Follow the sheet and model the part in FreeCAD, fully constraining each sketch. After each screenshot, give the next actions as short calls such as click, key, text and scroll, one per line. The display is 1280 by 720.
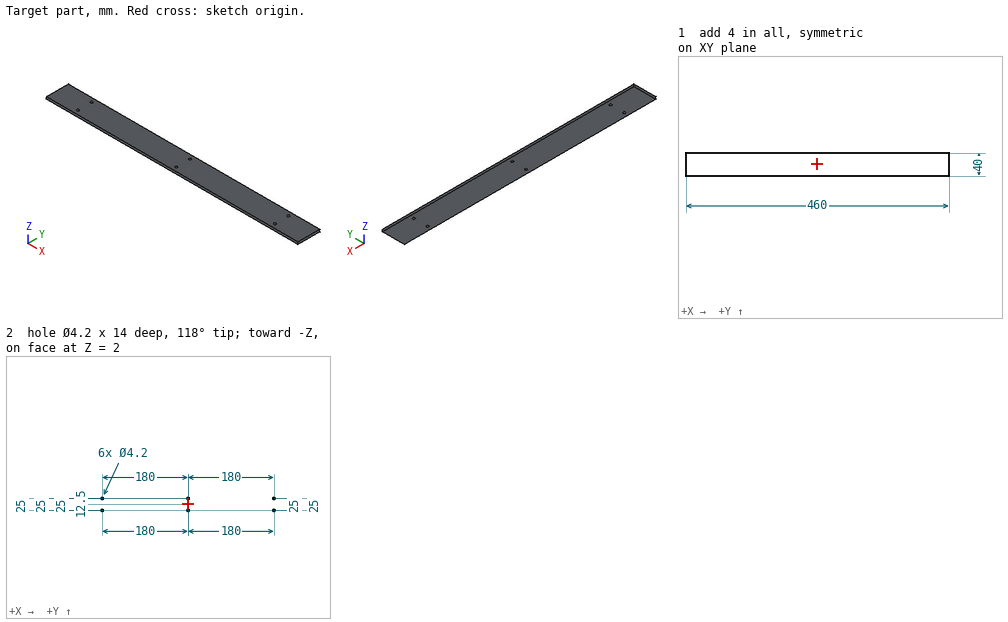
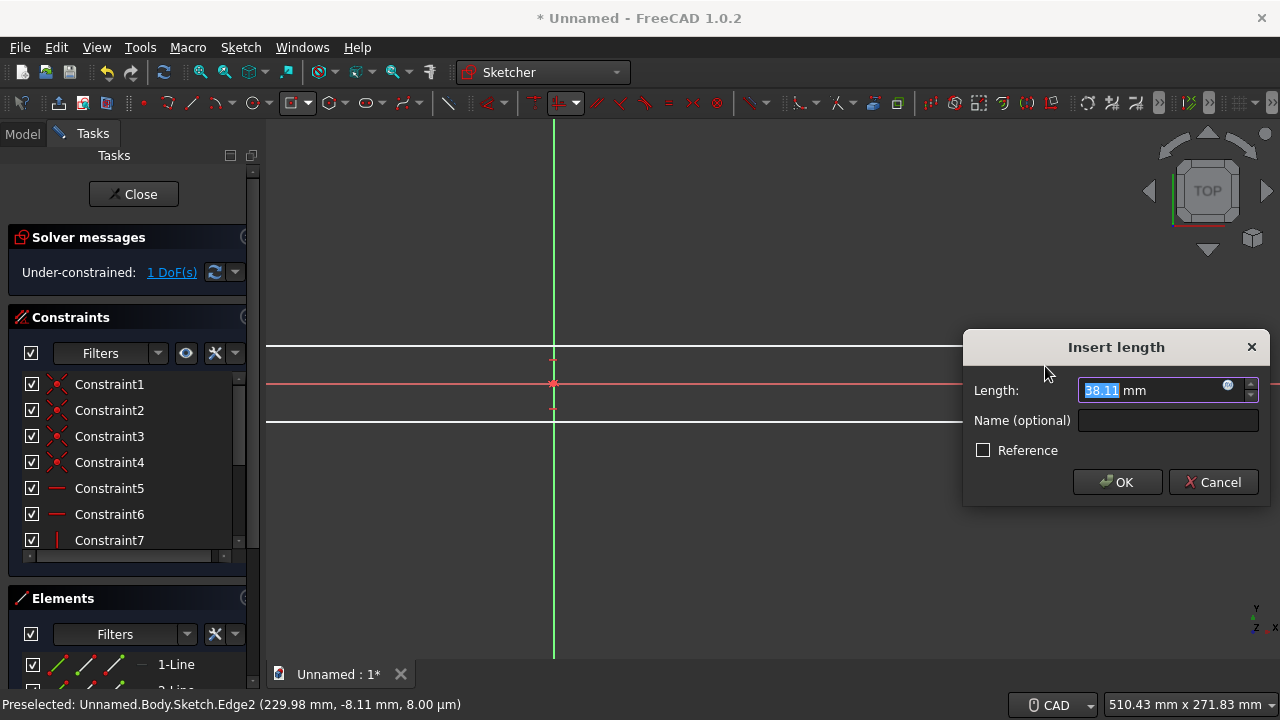
text(40)
key(Return)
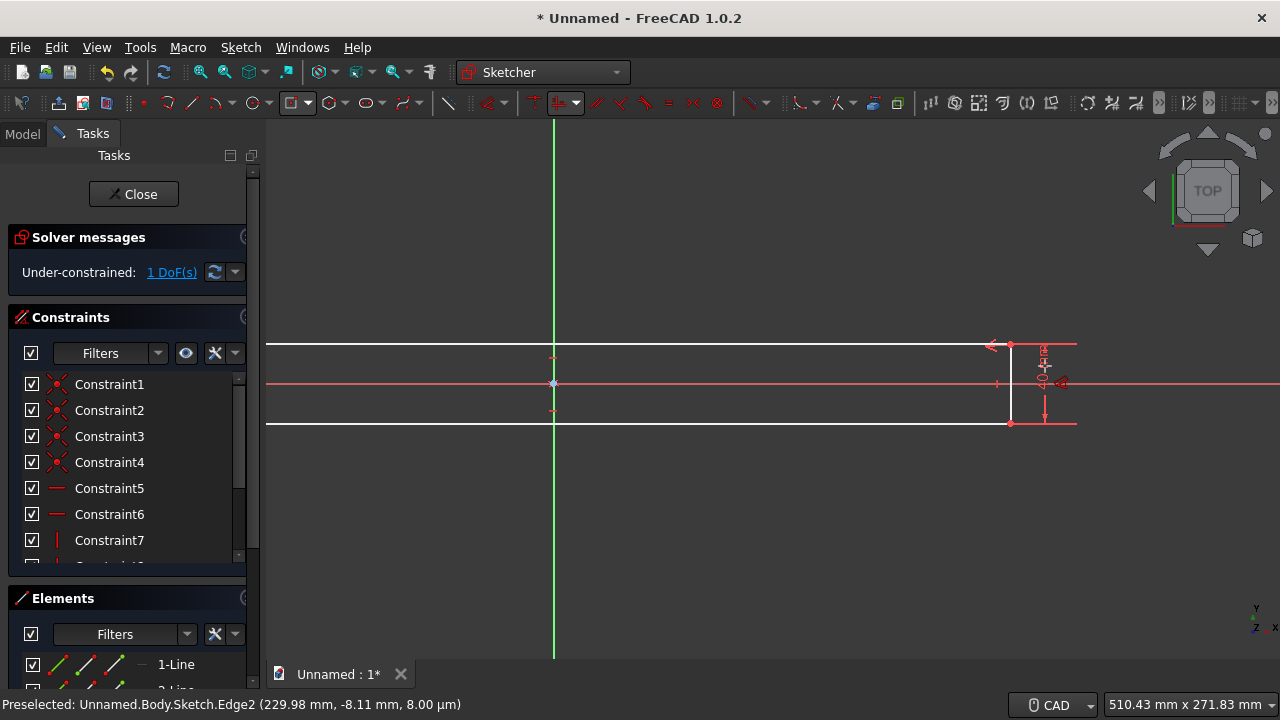
click(371, 424)
click(652, 458)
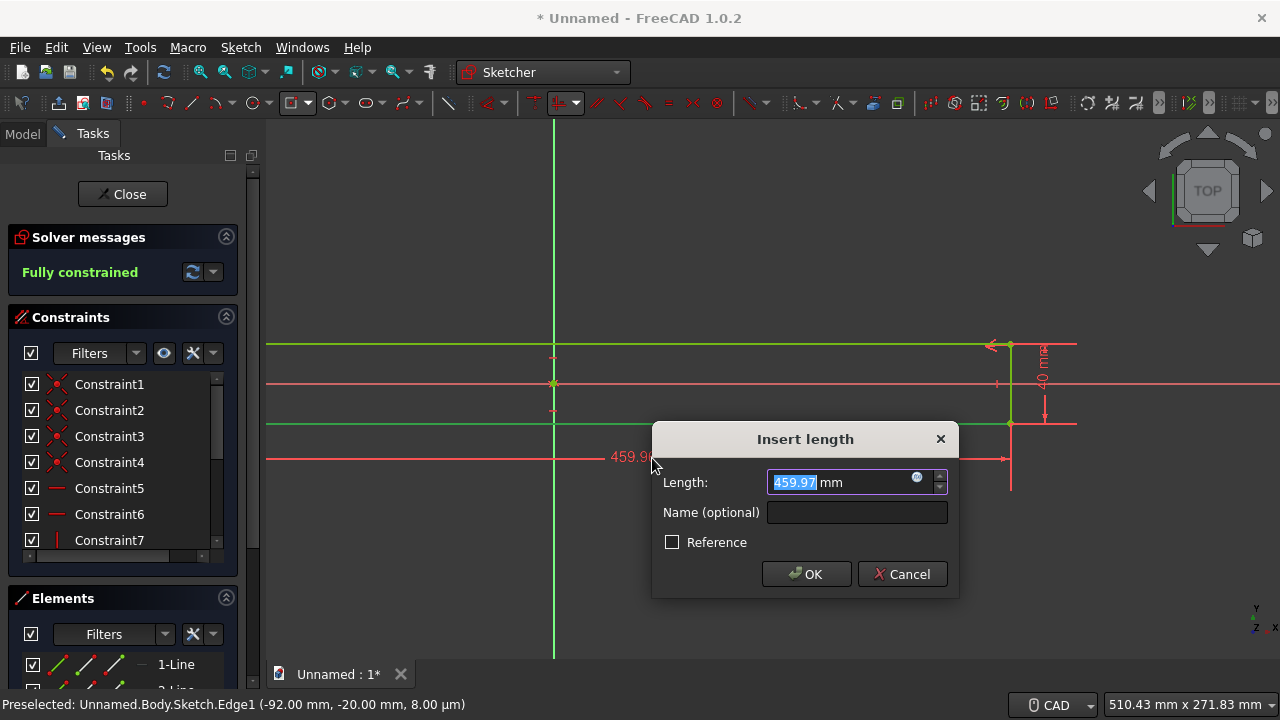
text(460)
key(Return)
key(Escape)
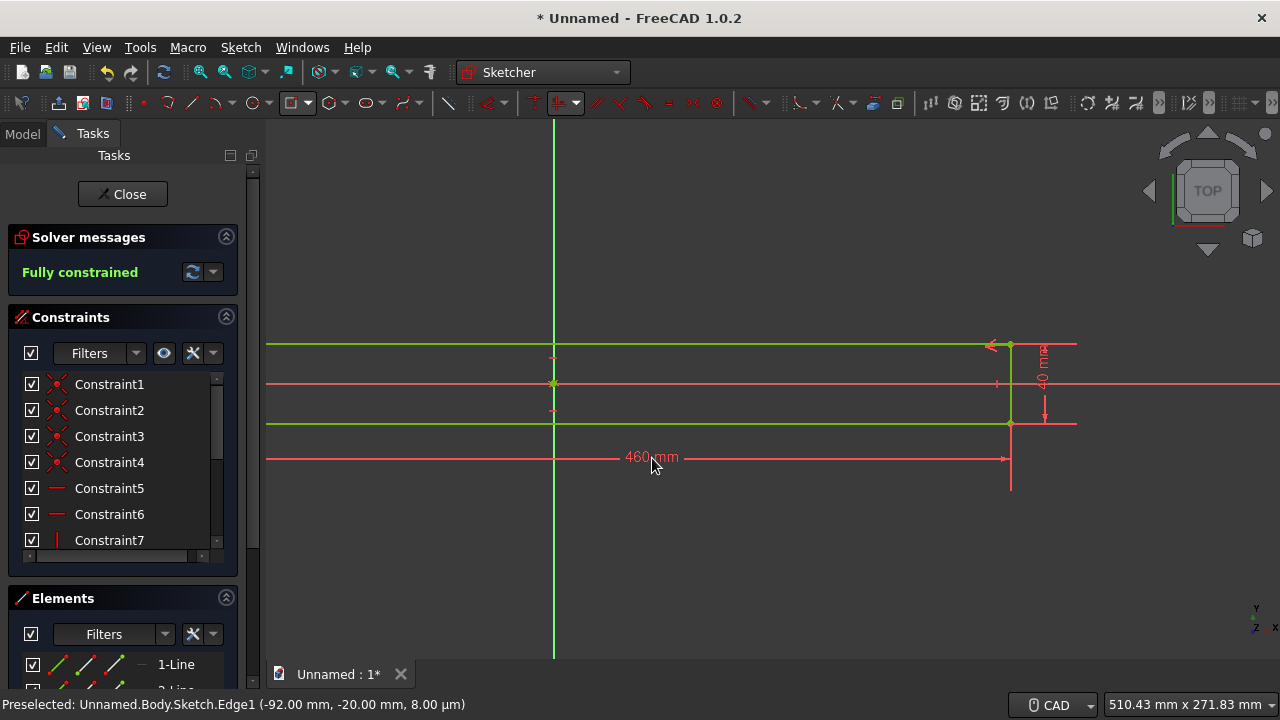
click(123, 194)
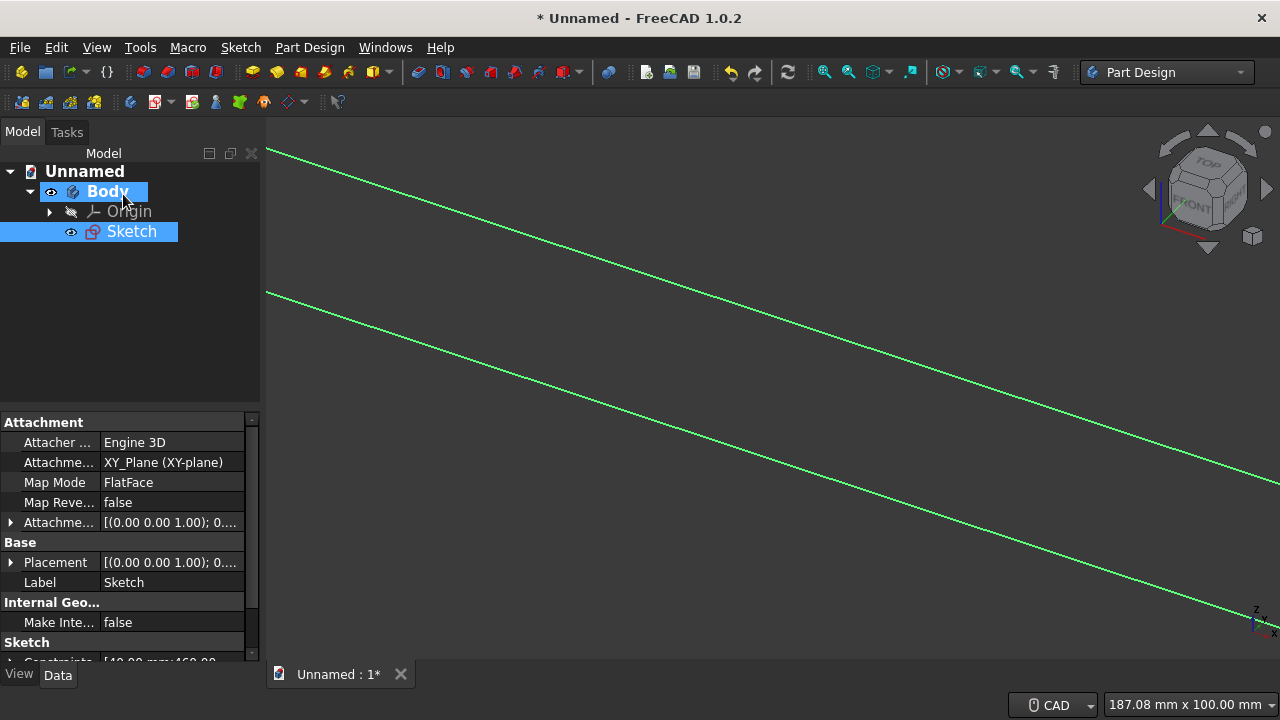
click(254, 72)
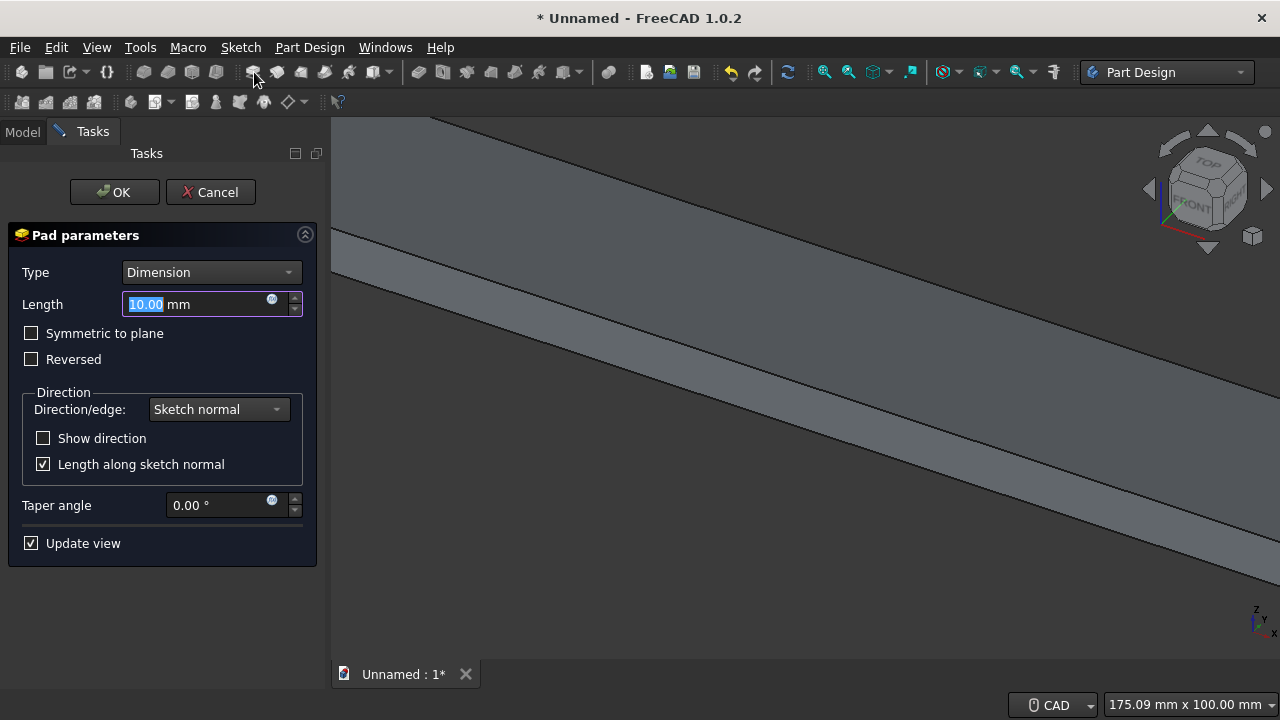
text(4)
key(Tab)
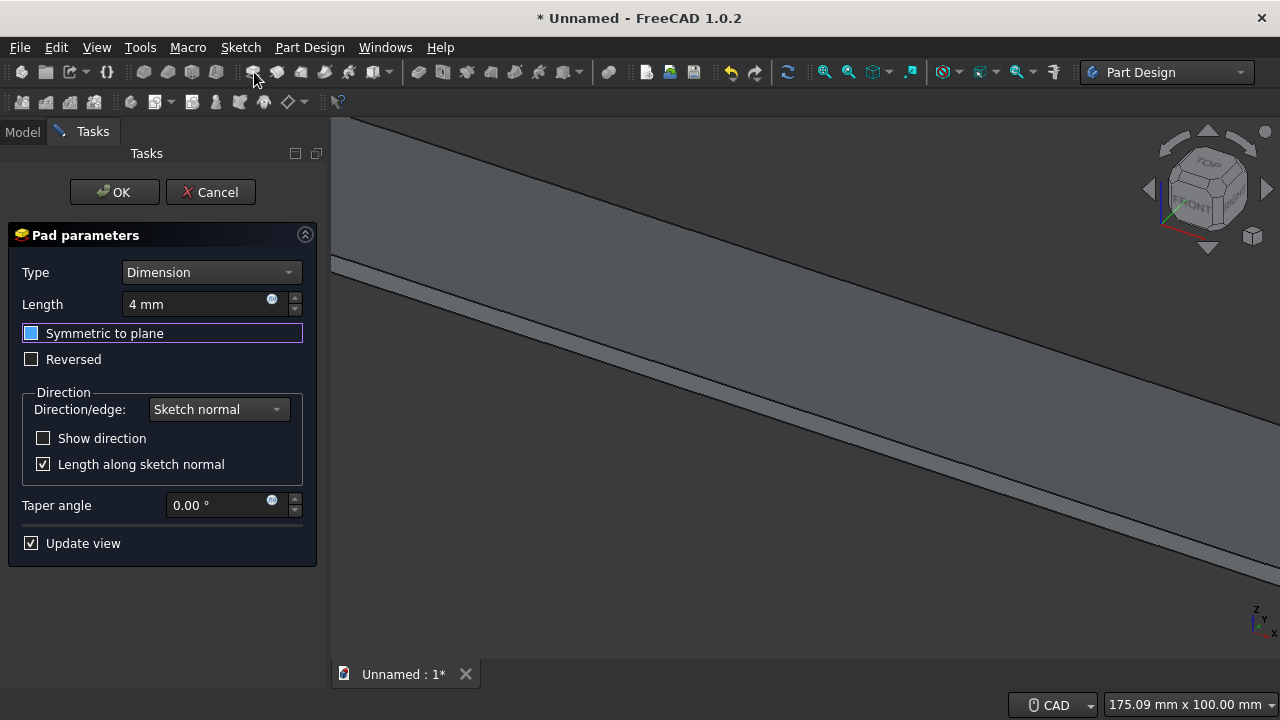
click(30, 333)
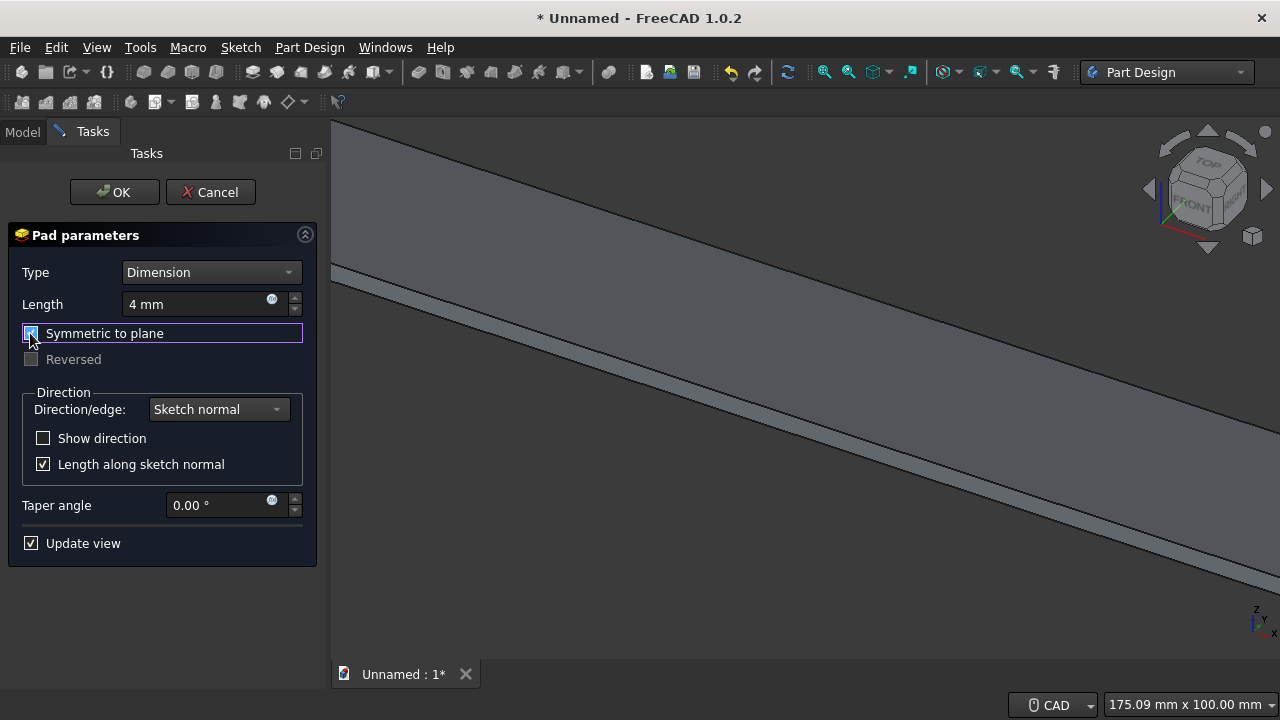
click(115, 192)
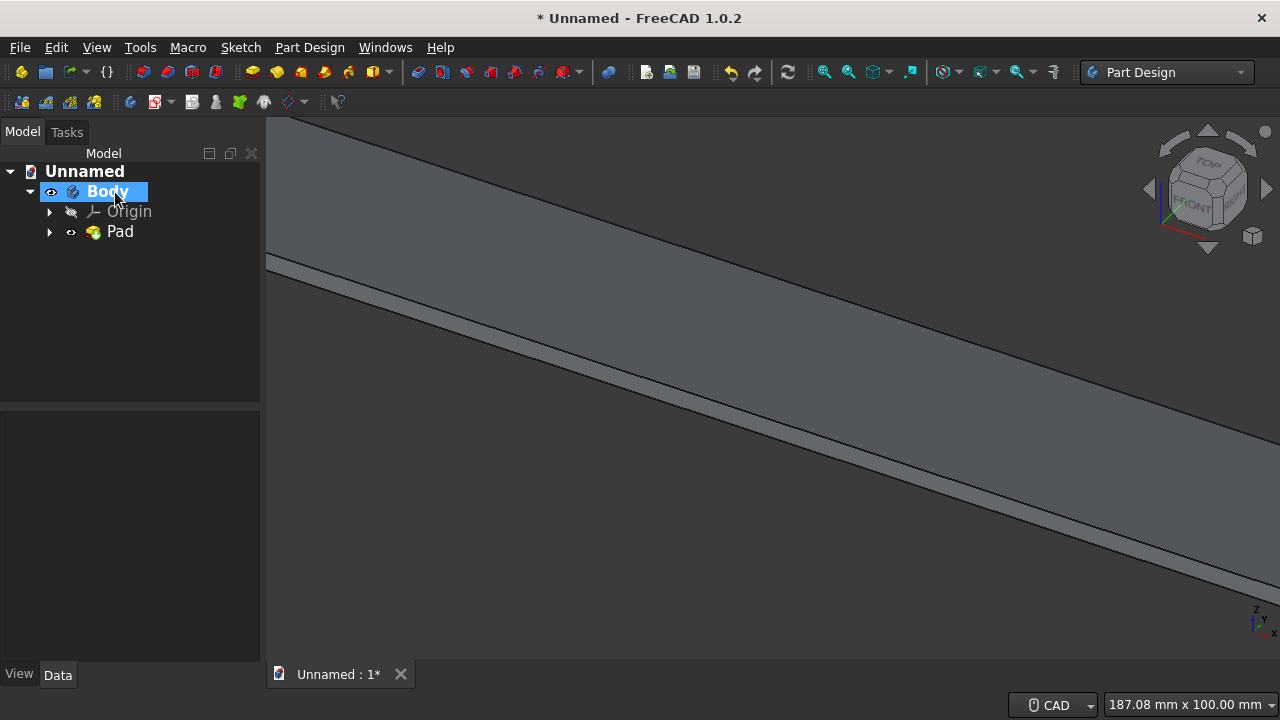
key(v)
key(f)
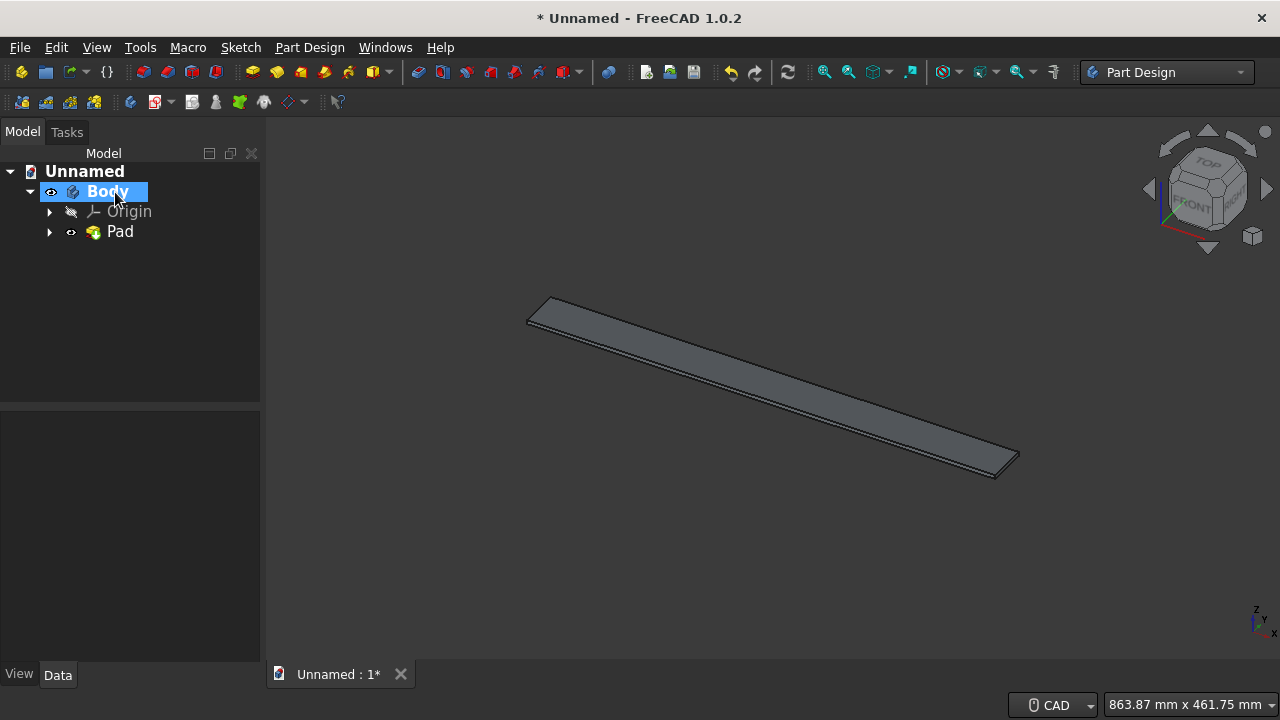
click(973, 451)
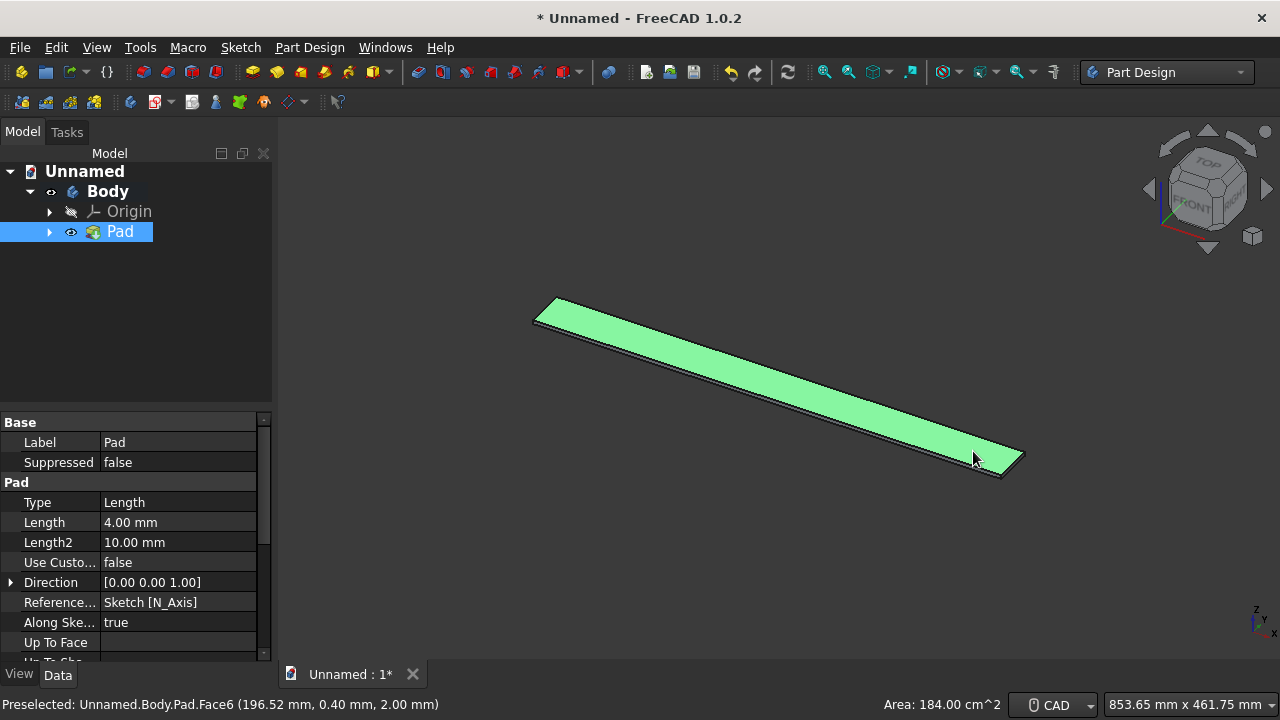
click(156, 102)